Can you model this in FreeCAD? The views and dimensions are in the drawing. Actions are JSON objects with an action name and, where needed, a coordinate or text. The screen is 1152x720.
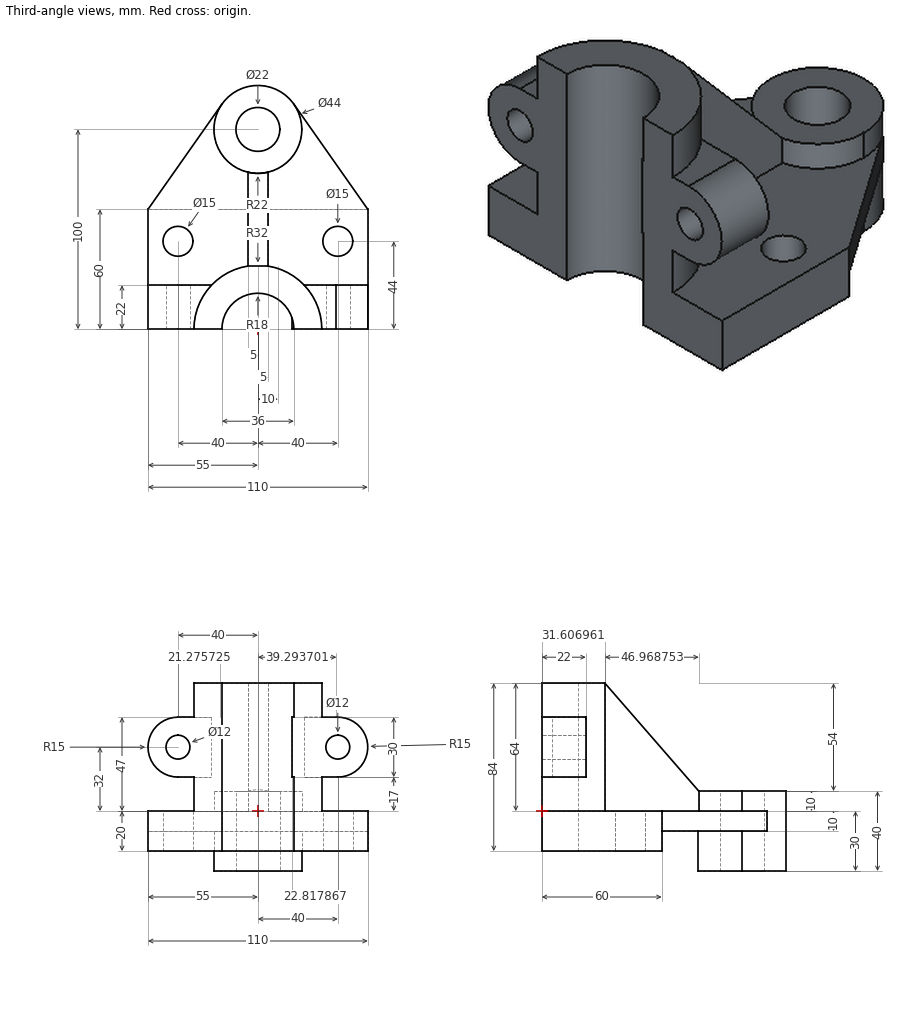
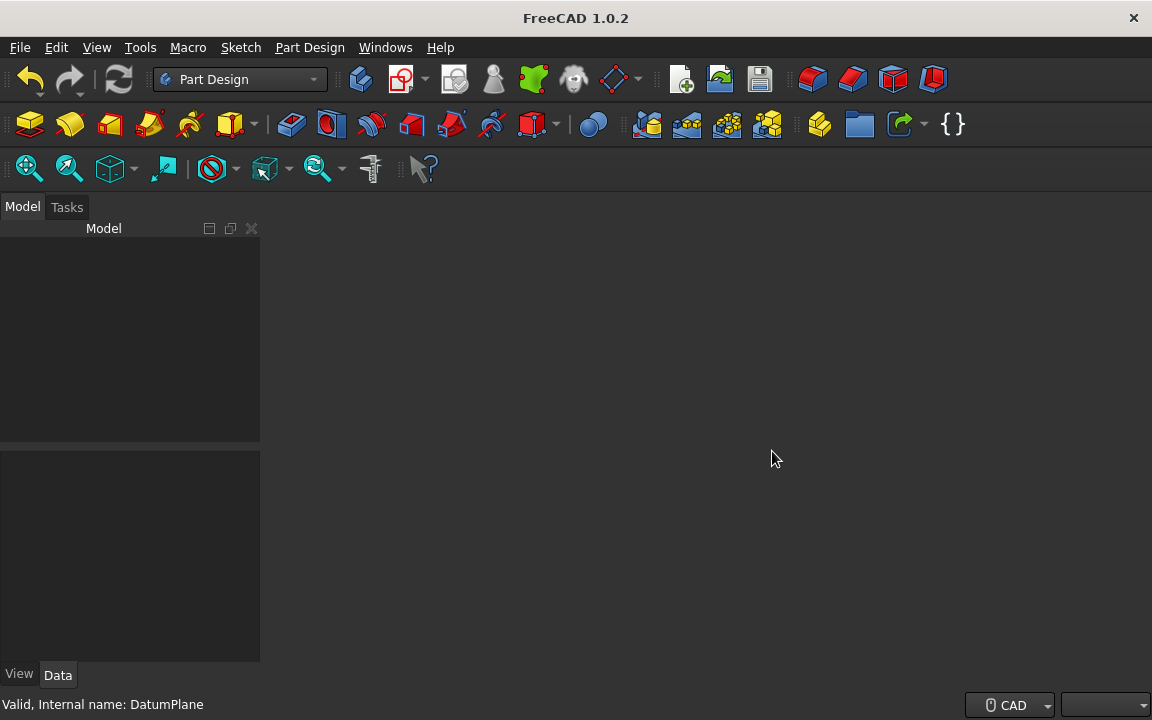
{"action": "left_click", "coordinate": [680, 80]}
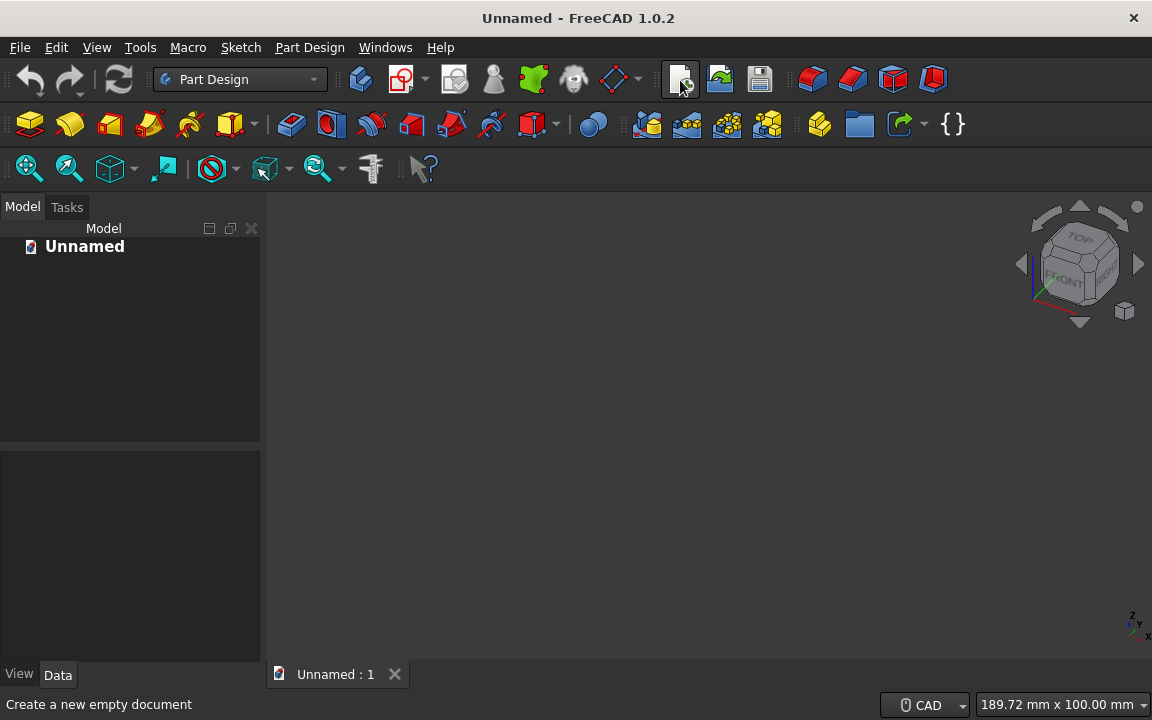
{"action": "left_click", "coordinate": [402, 80]}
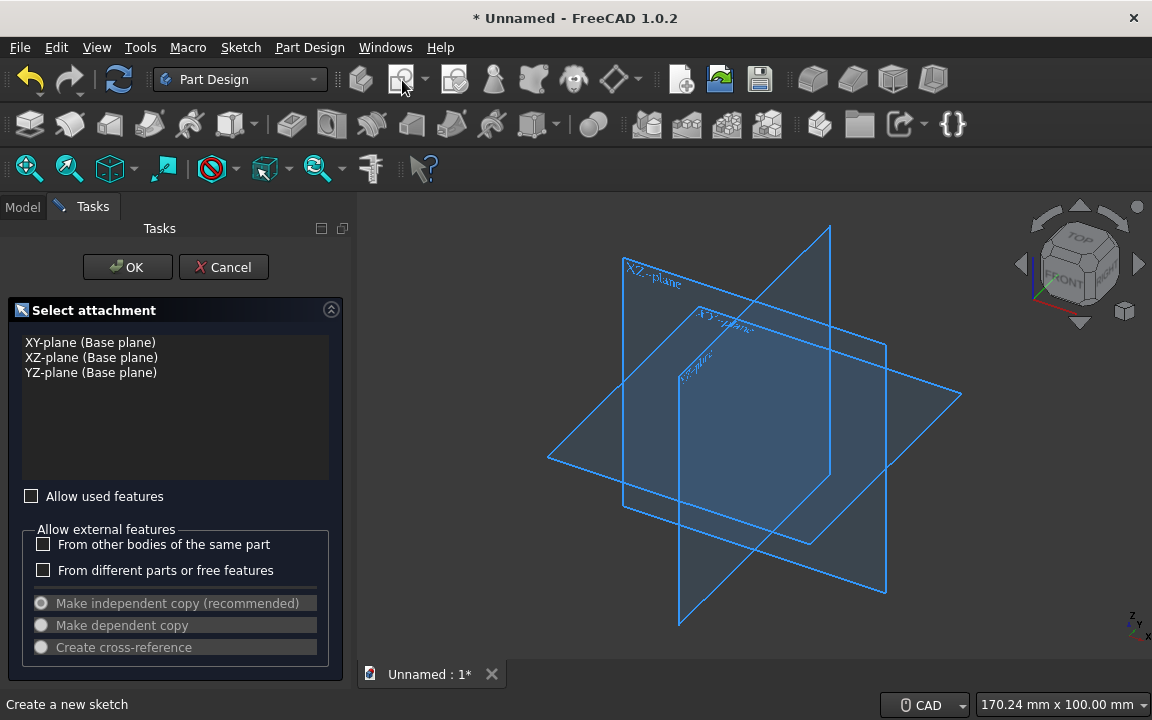
{"action": "left_click", "coordinate": [82, 358]}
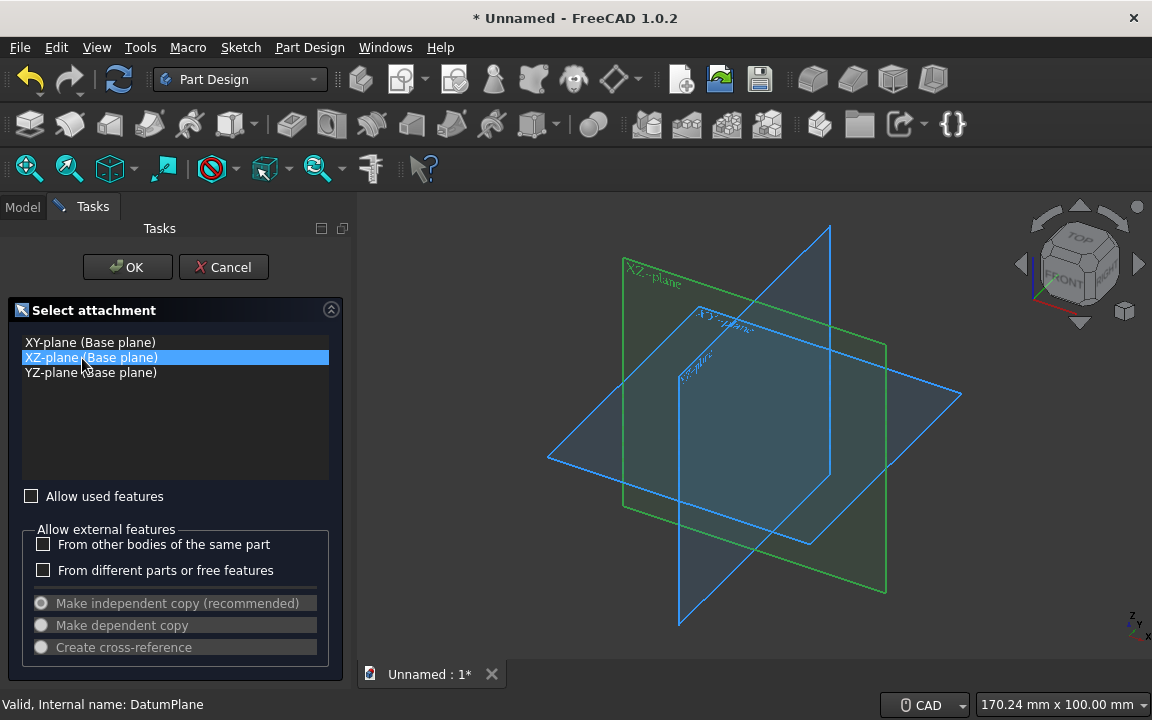
{"action": "left_click", "coordinate": [128, 267]}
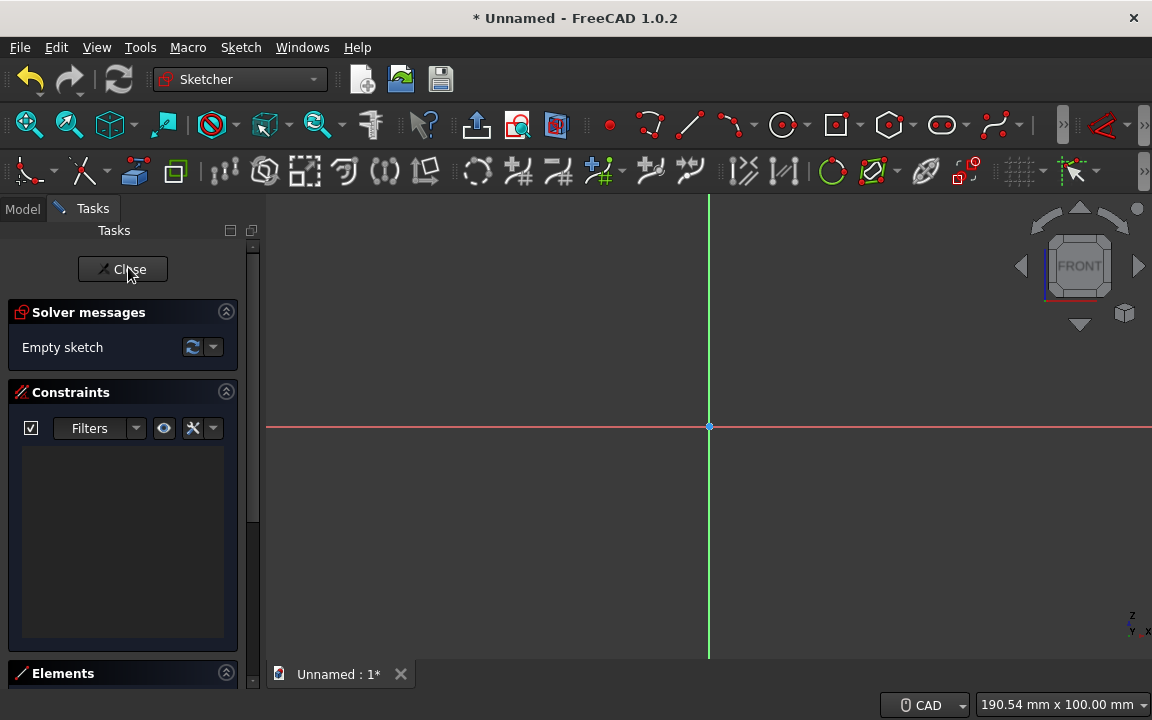
{"action": "scroll", "coordinate": [331, 222], "scroll_direction": "down", "scroll_amount": 1}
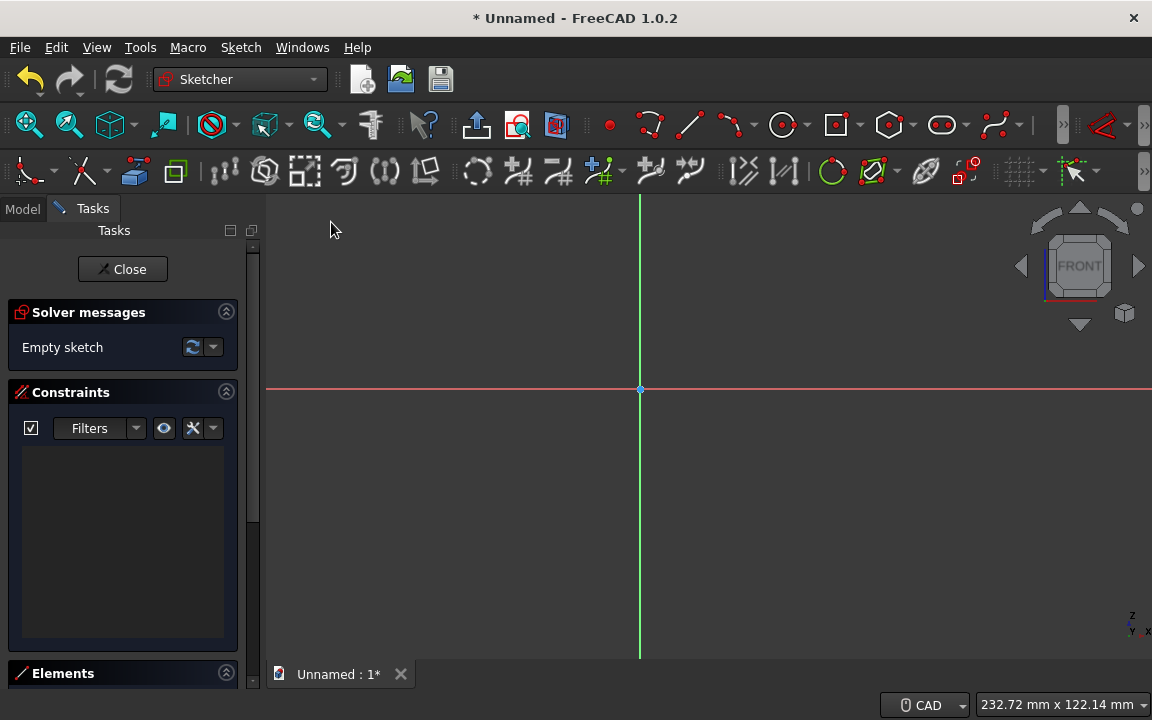
{"action": "left_click", "coordinate": [862, 126]}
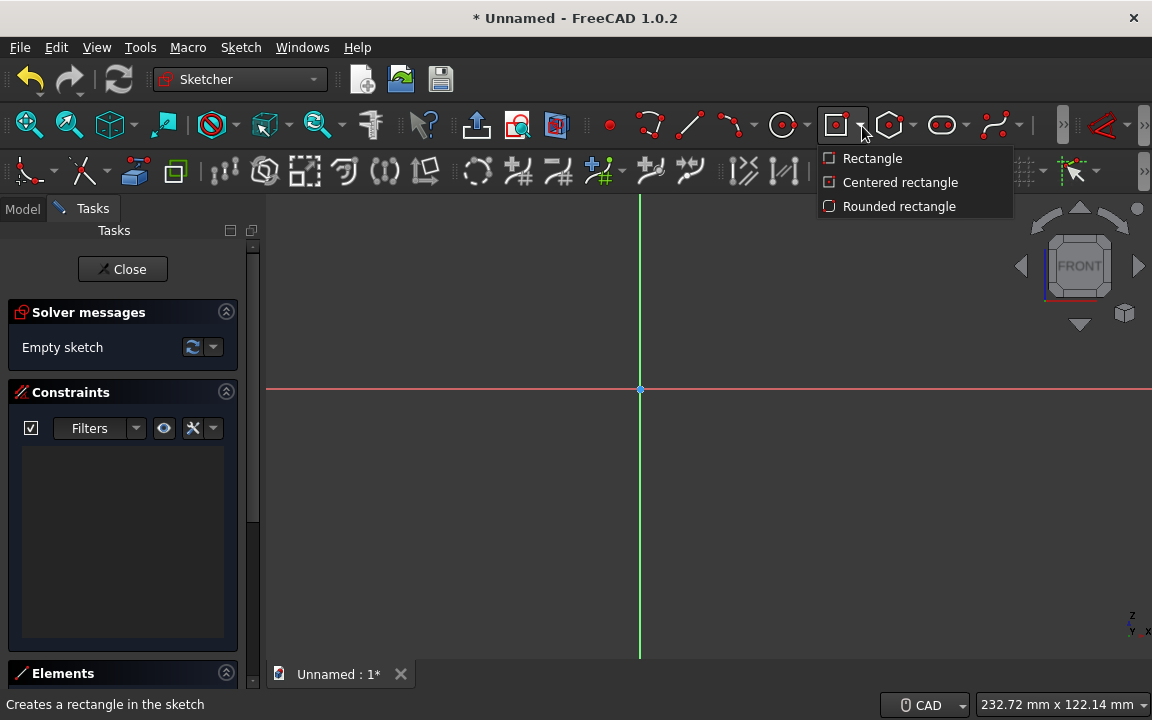
{"action": "left_click", "coordinate": [916, 158]}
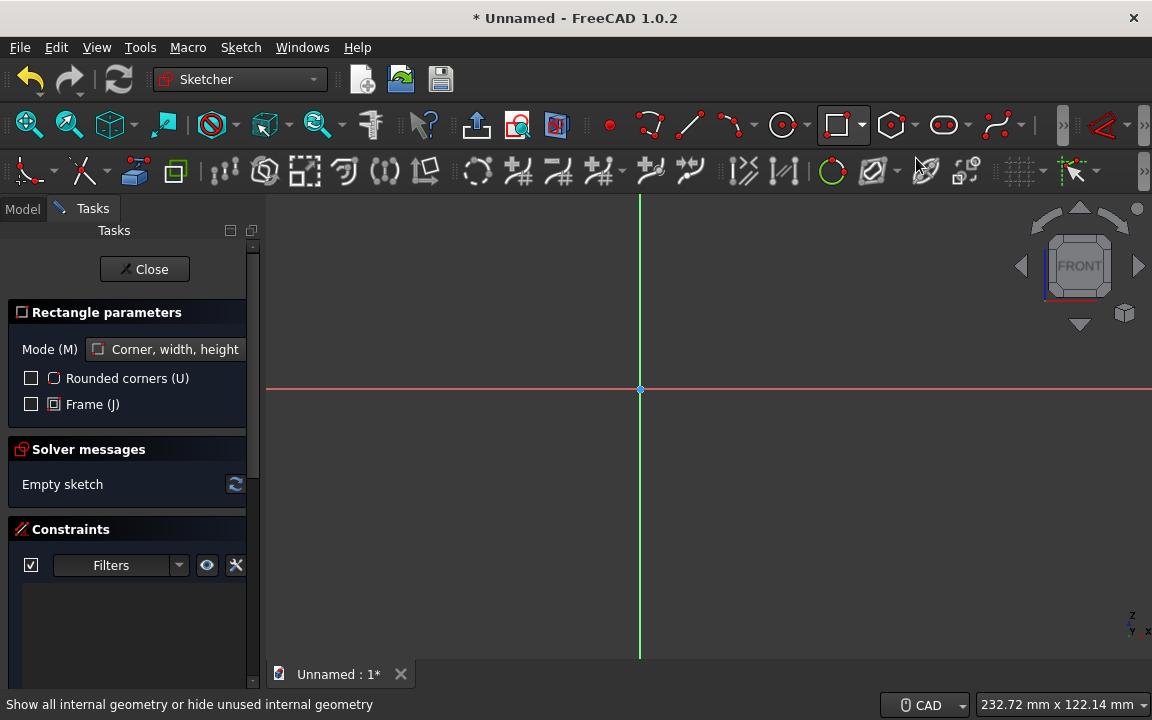
{"action": "left_click", "coordinate": [431, 389]}
{"action": "left_click", "coordinate": [850, 466]}
{"action": "key", "text": "Escape"}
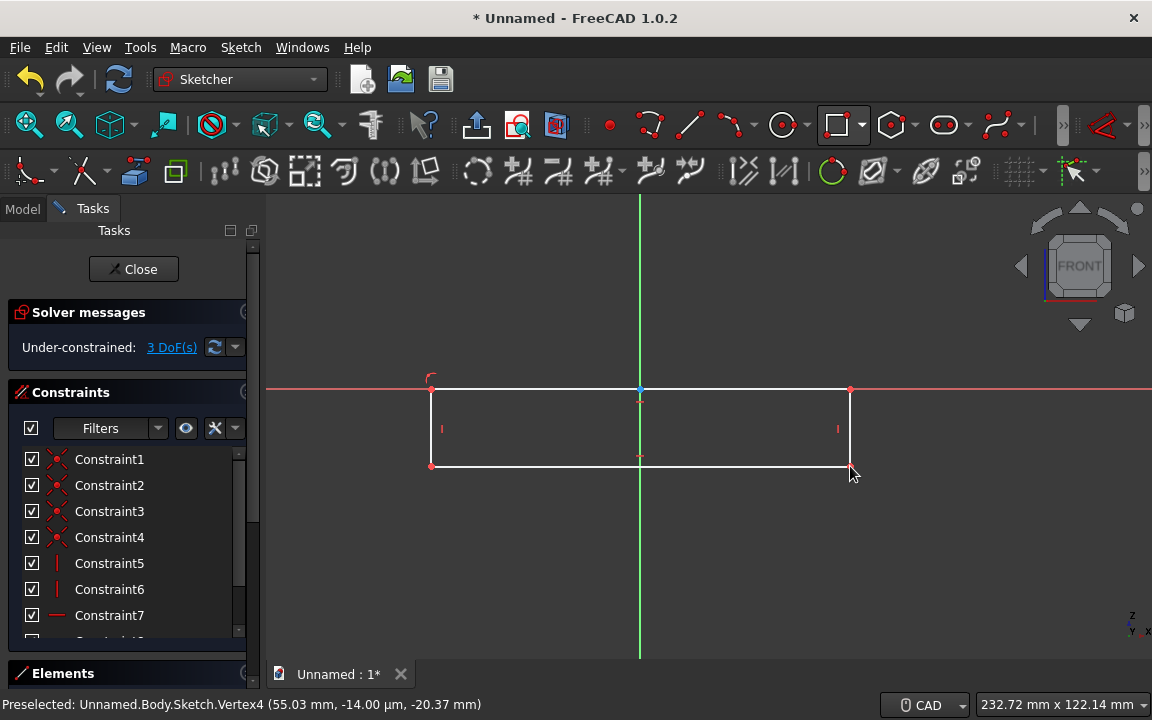
{"action": "left_click", "coordinate": [1102, 126]}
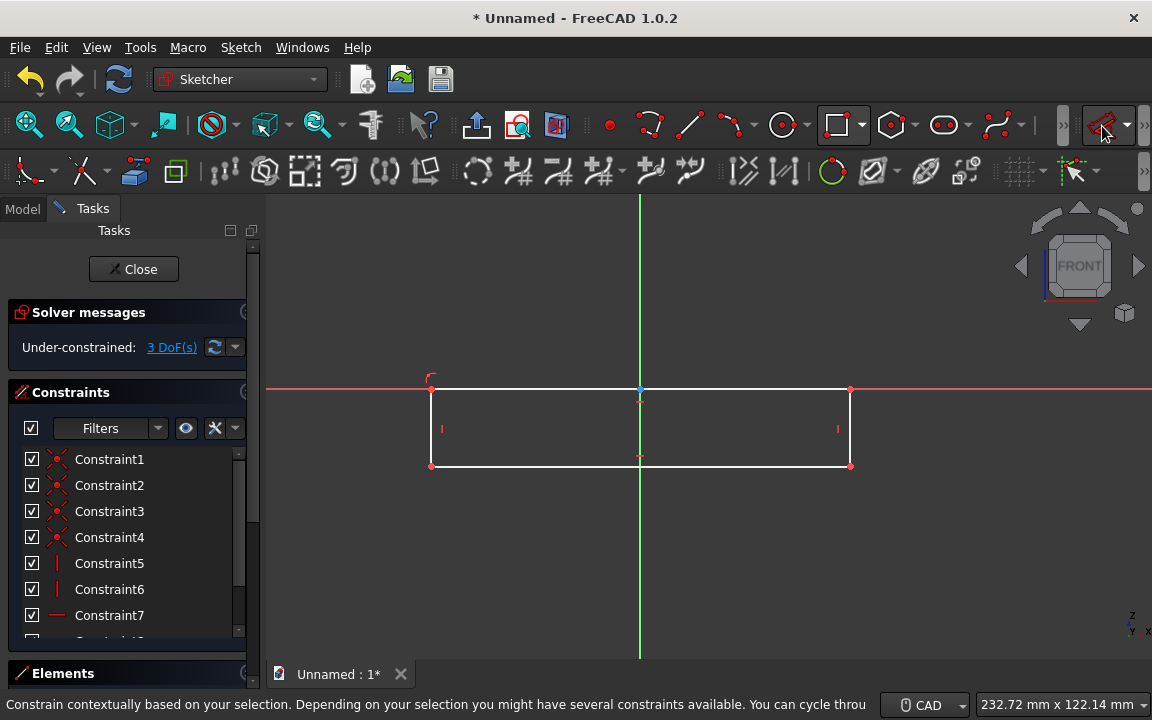
{"action": "left_click", "coordinate": [431, 413]}
{"action": "left_click", "coordinate": [397, 428]}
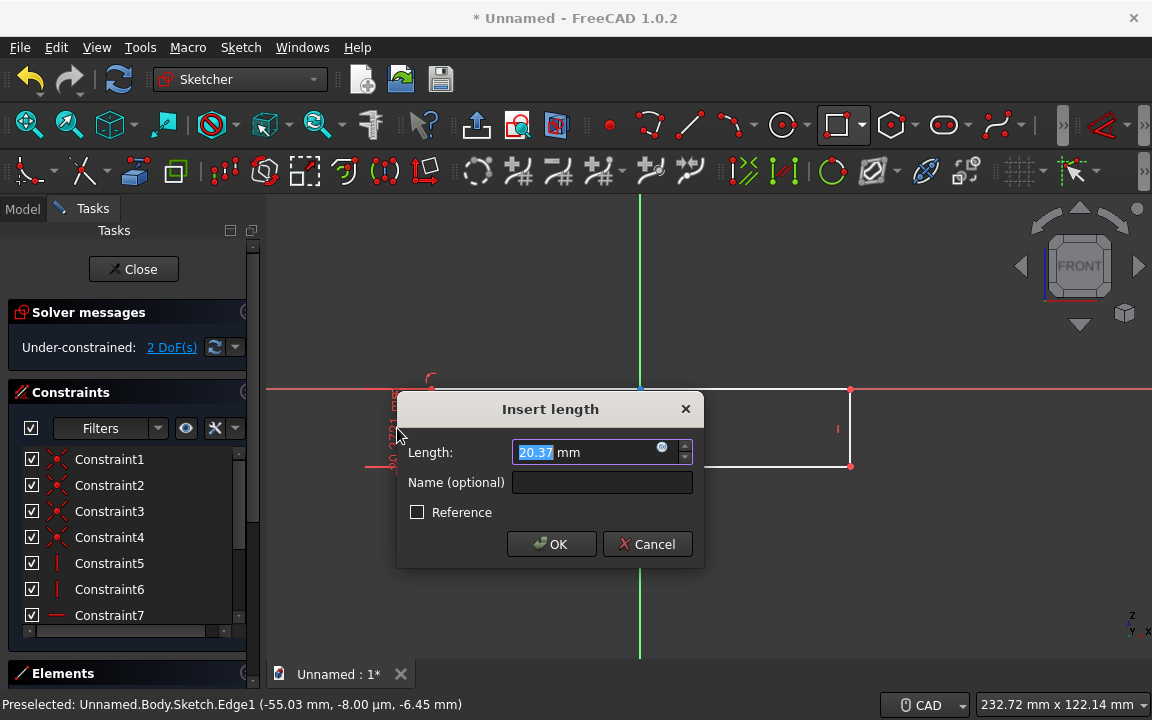
{"action": "type", "text": "20"}
{"action": "key", "text": "Return"}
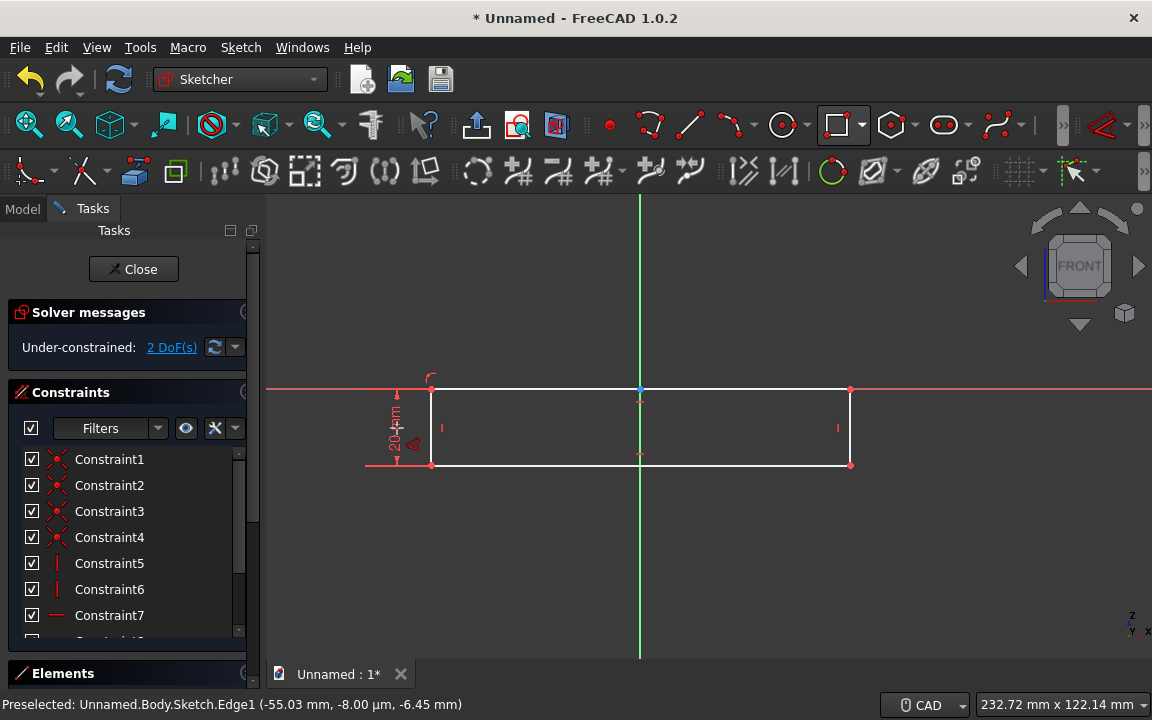
{"action": "left_click", "coordinate": [557, 466]}
{"action": "left_click", "coordinate": [544, 500]}